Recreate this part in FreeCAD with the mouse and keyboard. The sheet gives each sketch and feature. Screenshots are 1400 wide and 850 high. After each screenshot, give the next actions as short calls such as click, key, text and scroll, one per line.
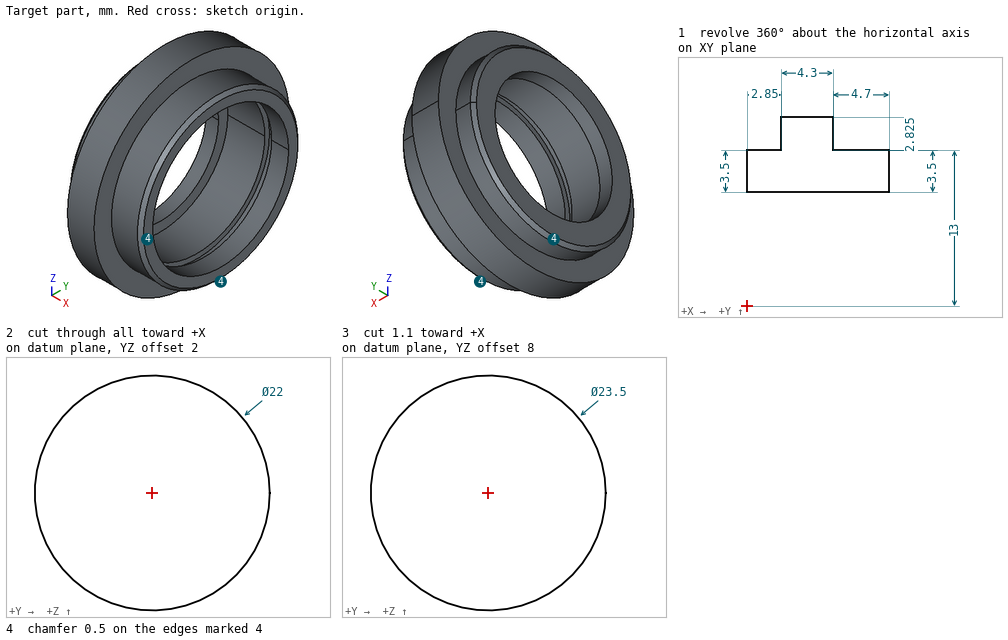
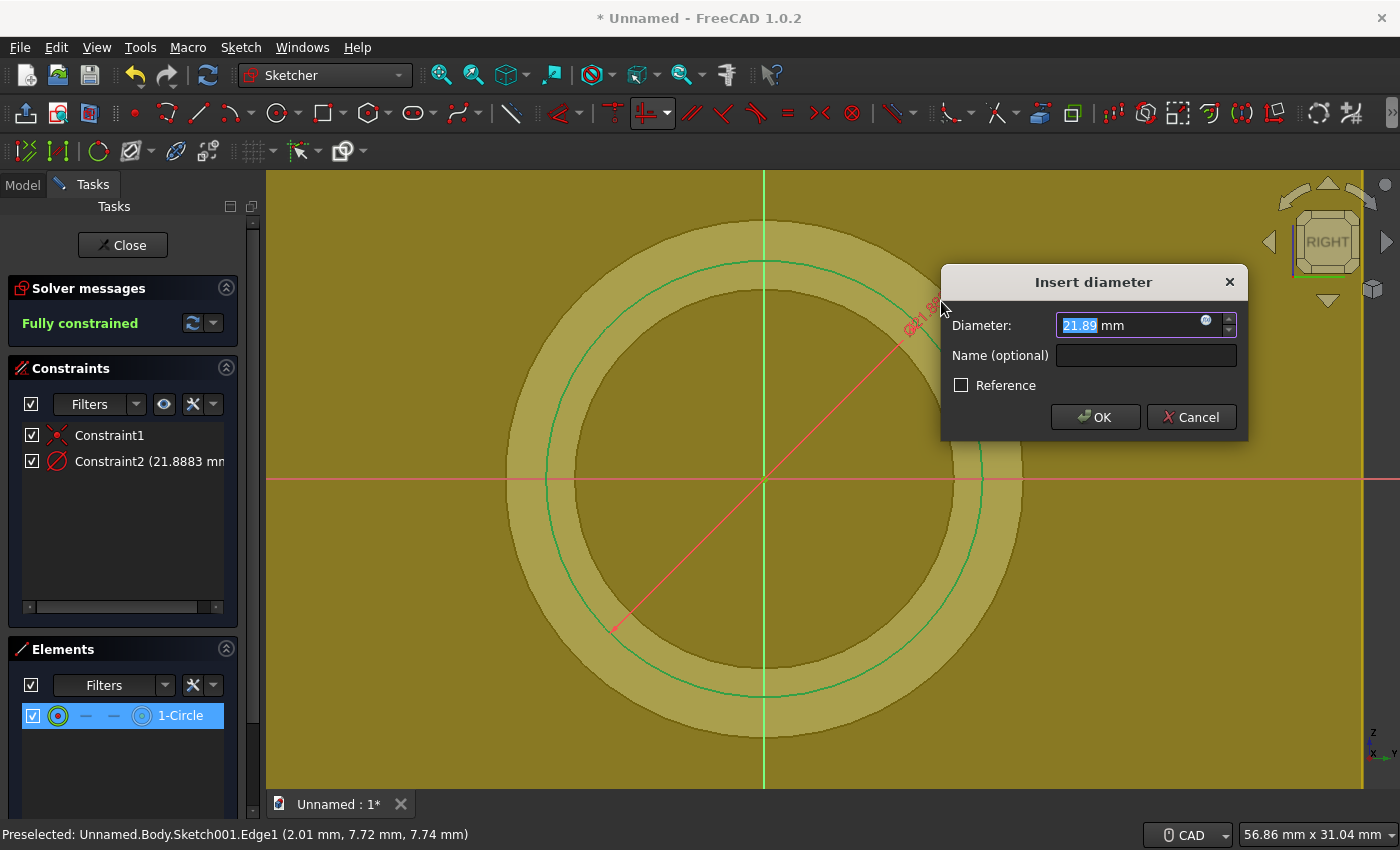
text(22)
key(Return)
key(Escape)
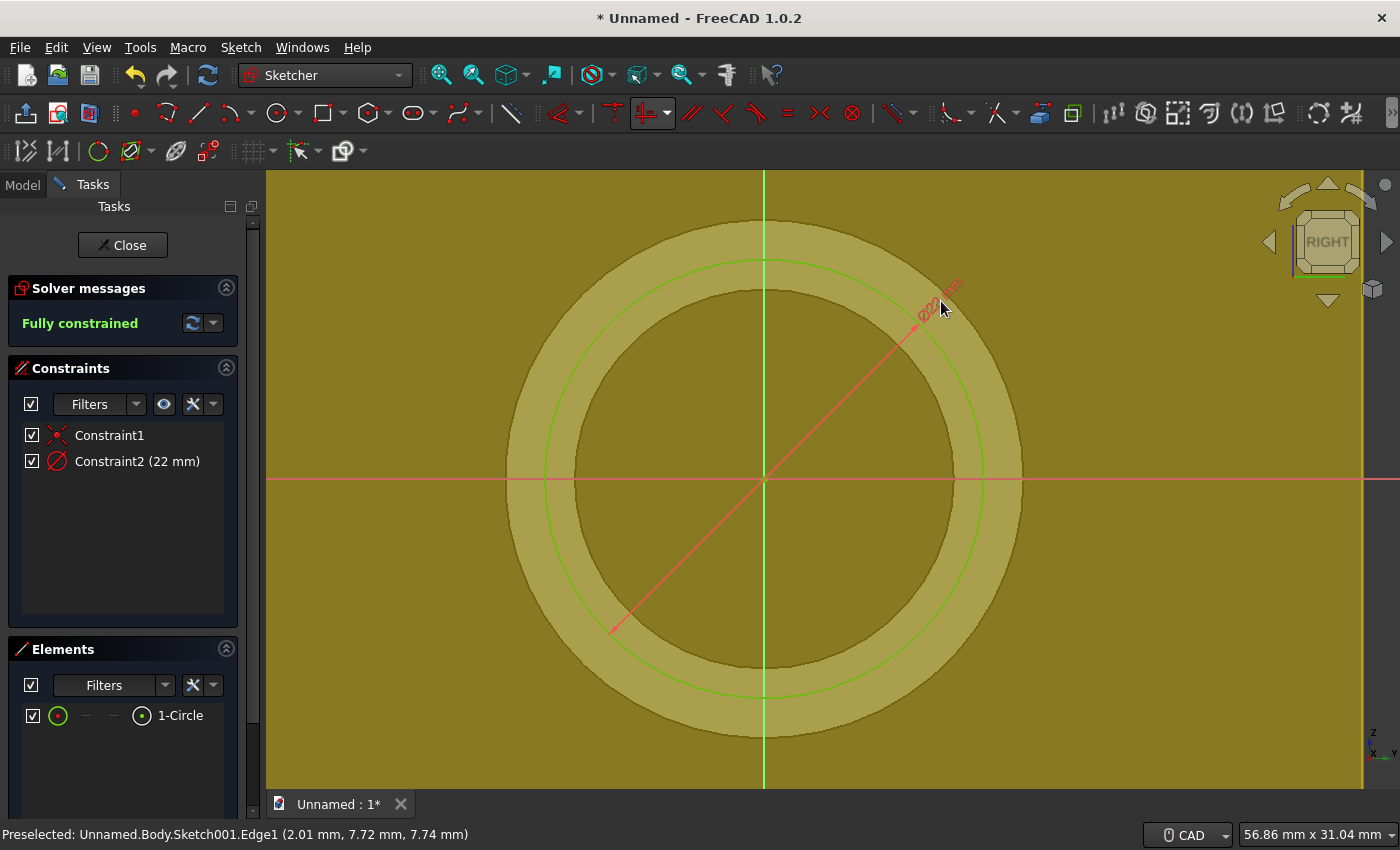
click(123, 245)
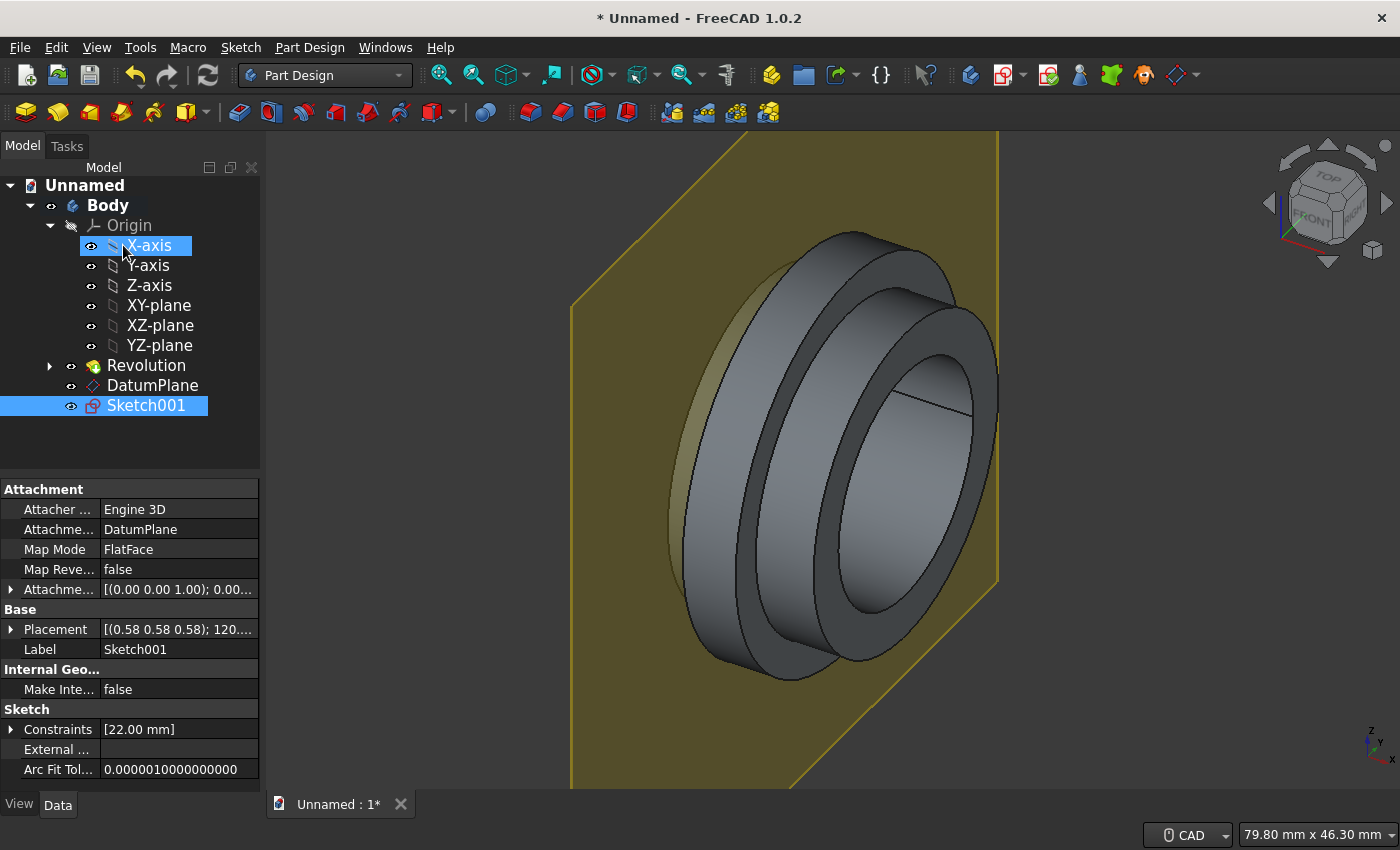
click(240, 112)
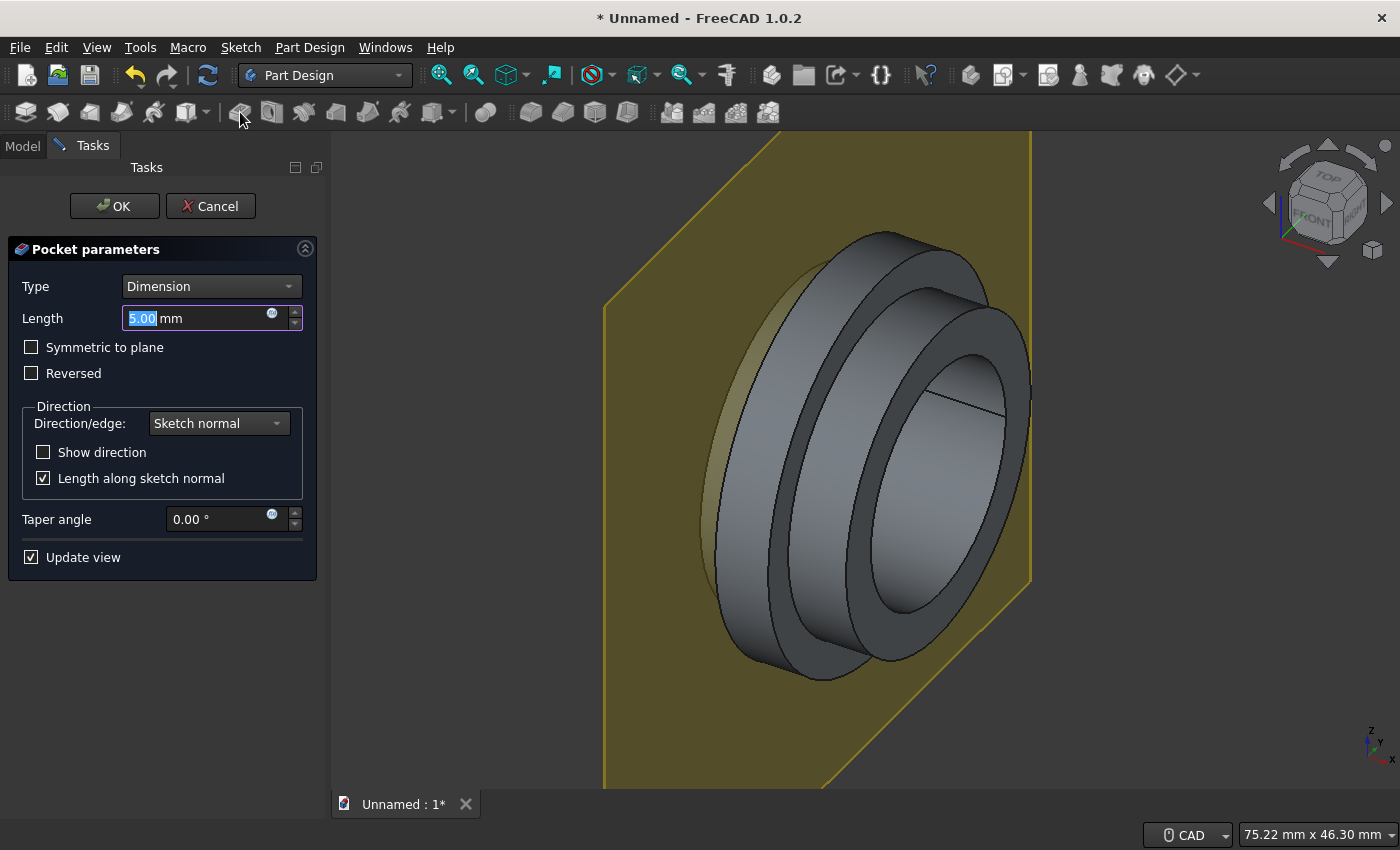
click(212, 286)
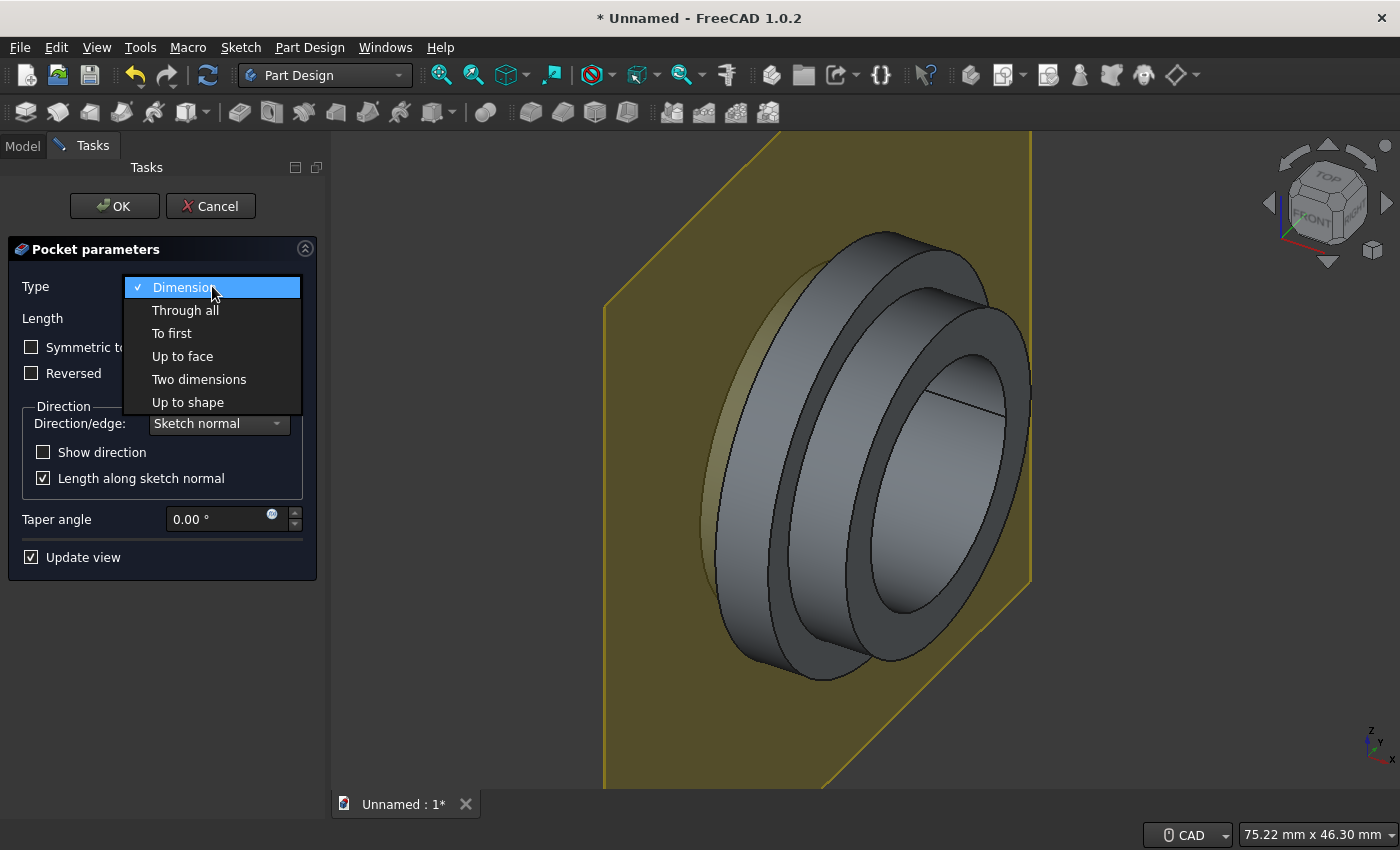
click(212, 310)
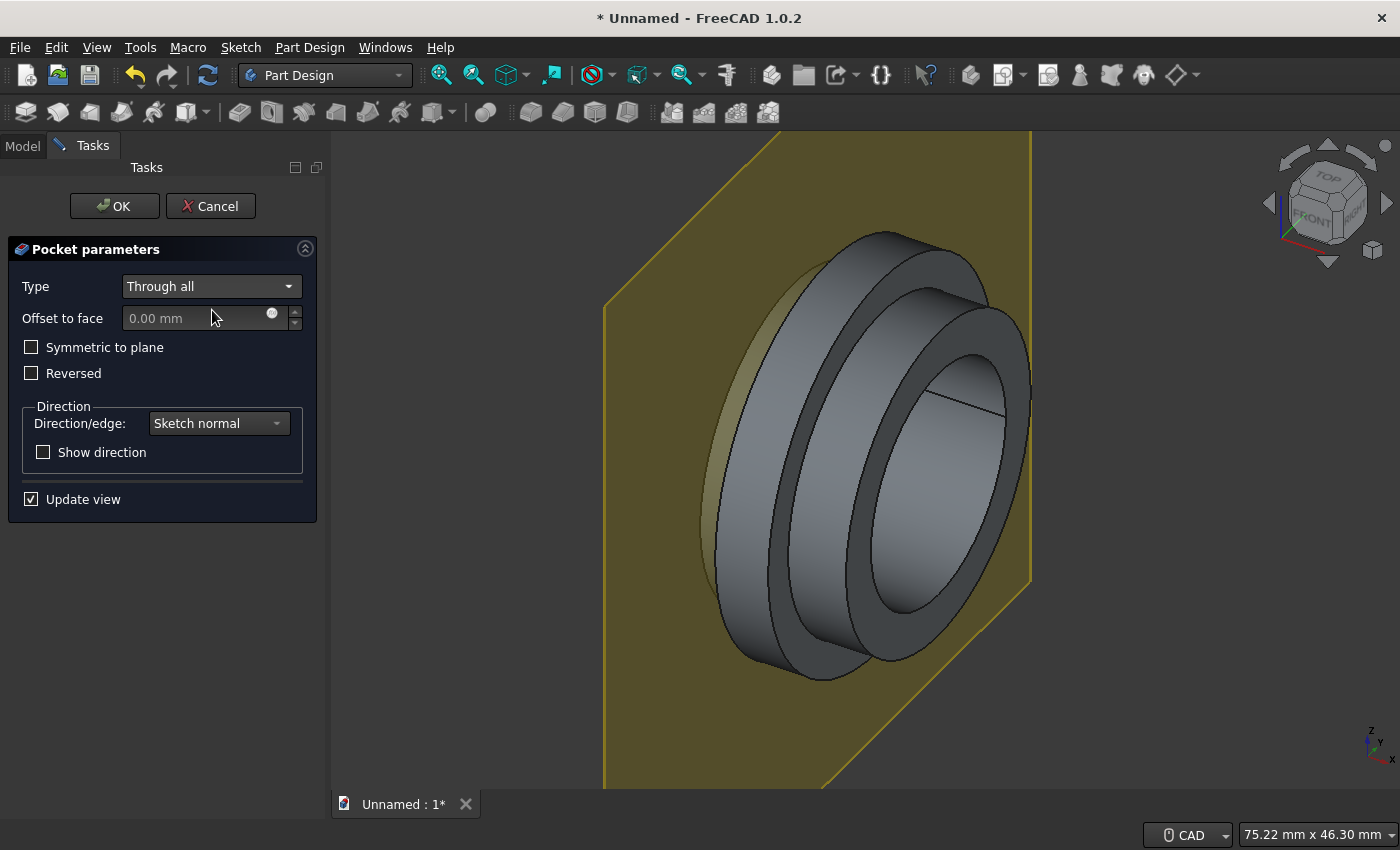
click(30, 373)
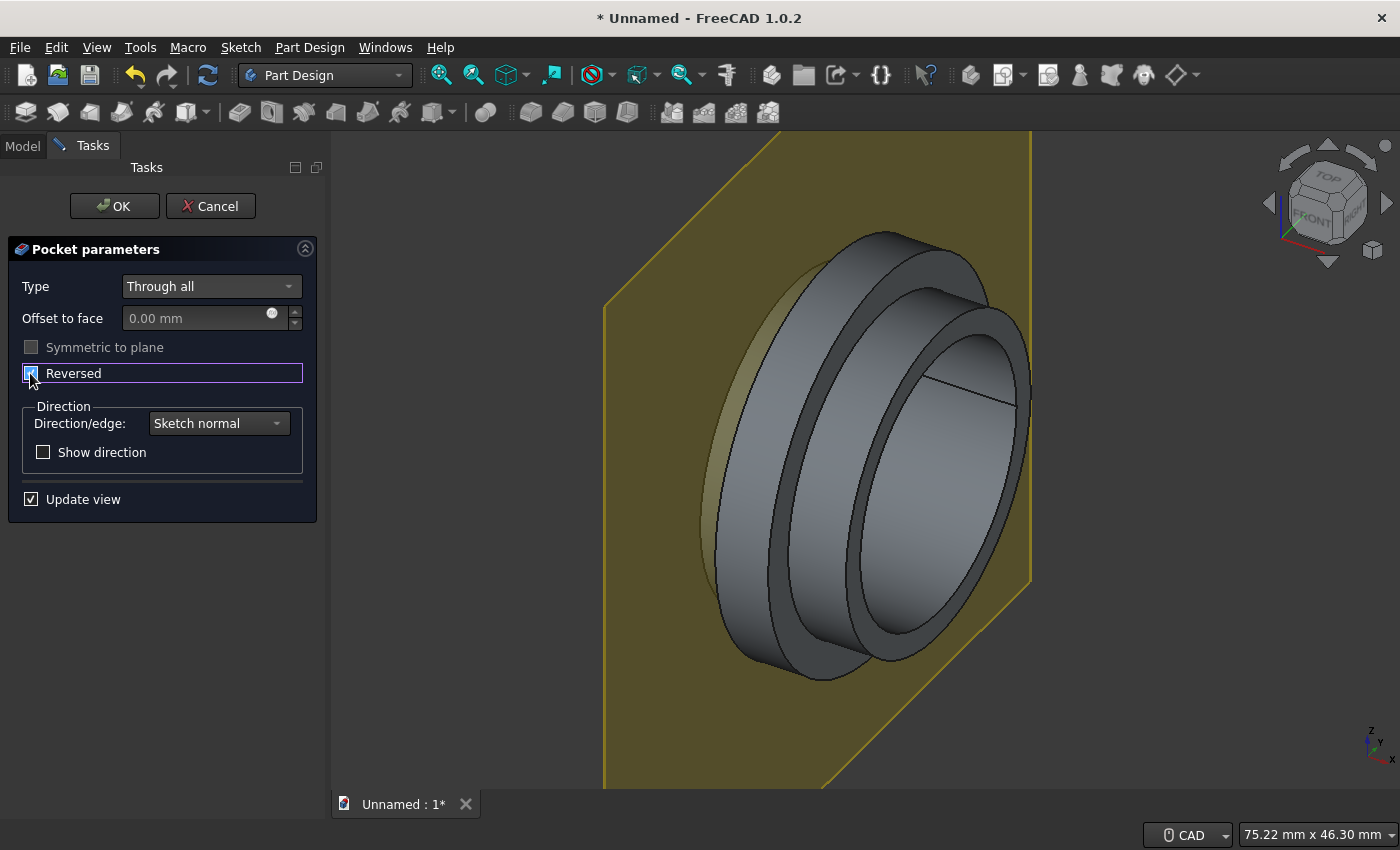
click(115, 206)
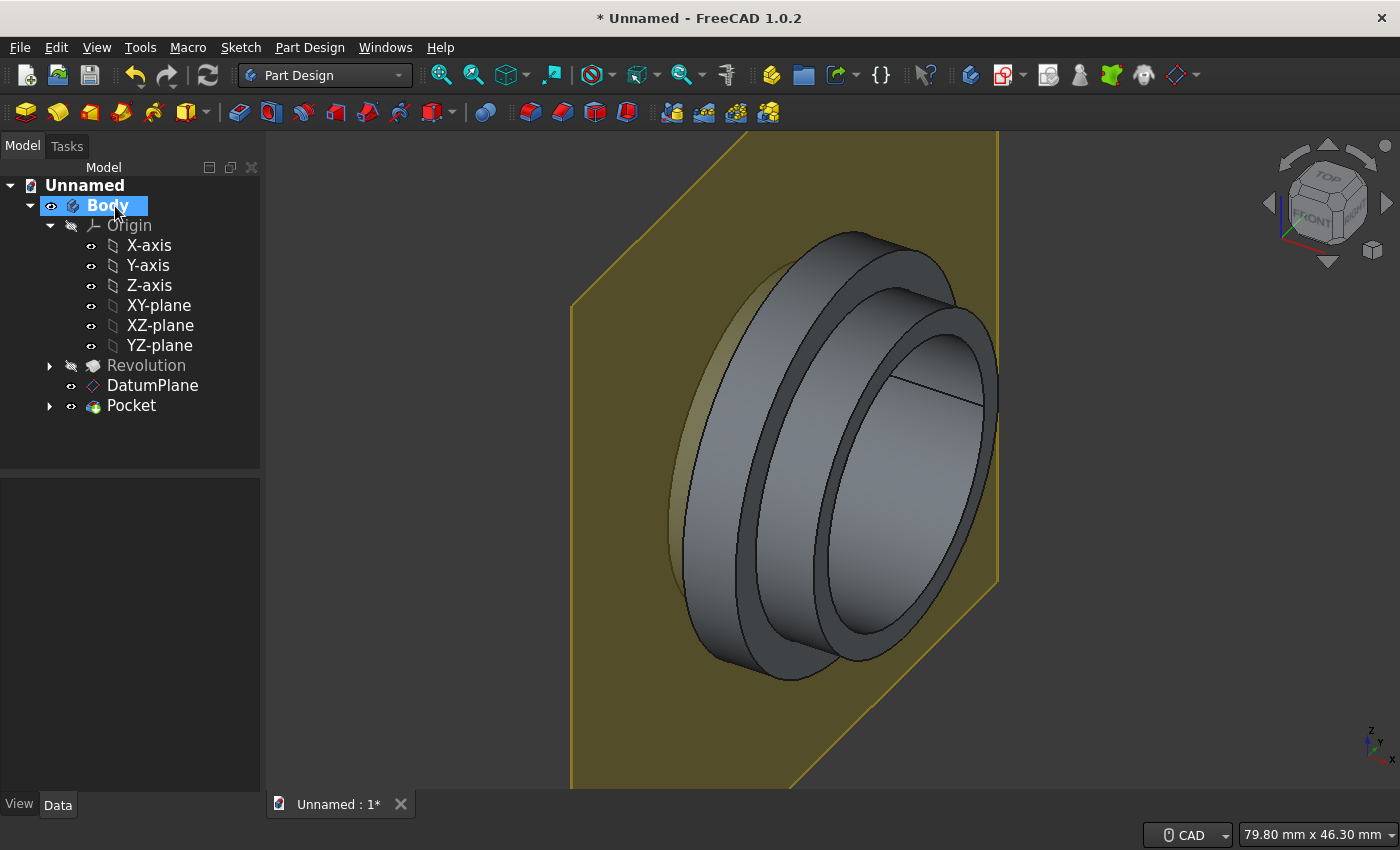
click(116, 386)
key(space)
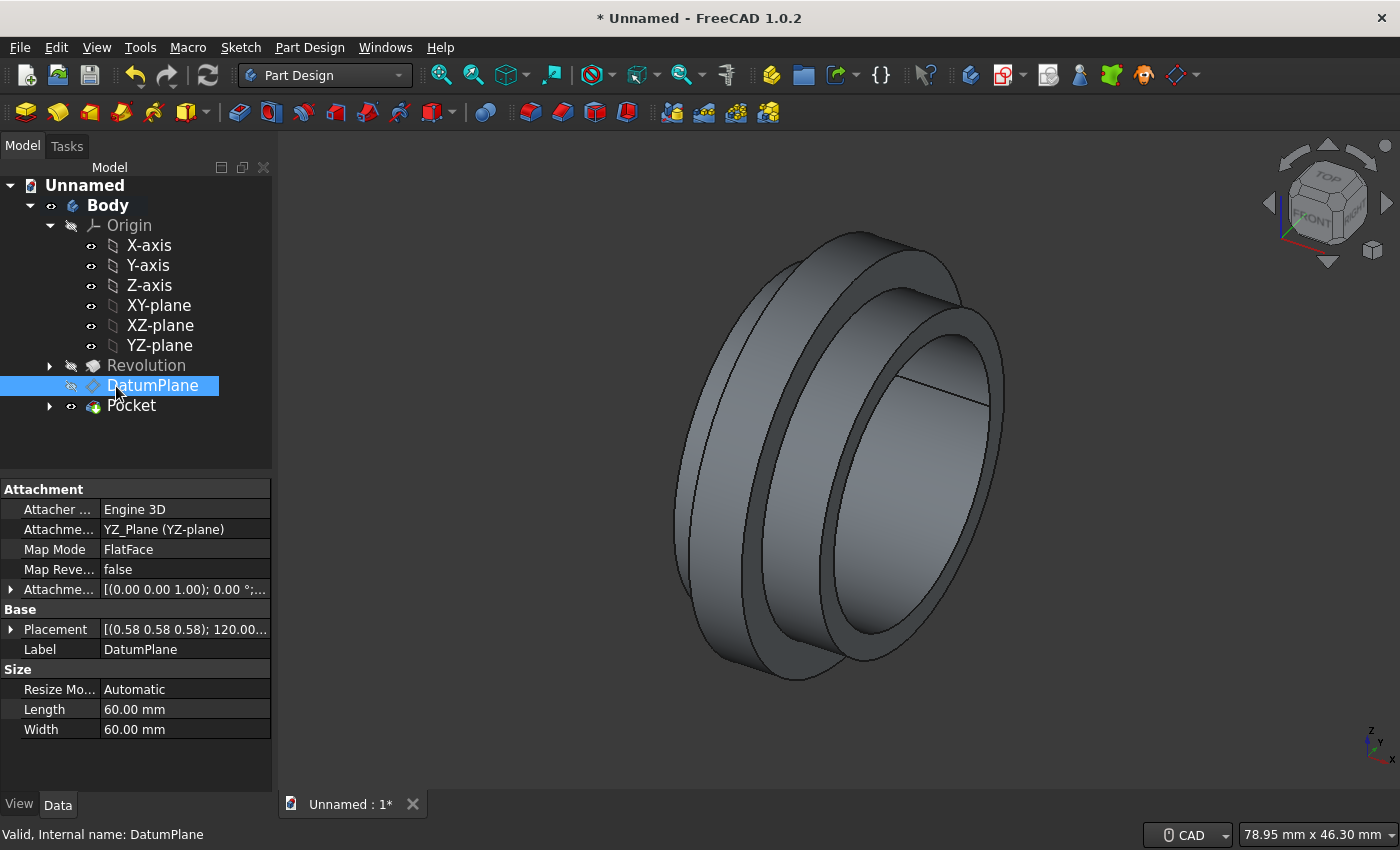
click(136, 346)